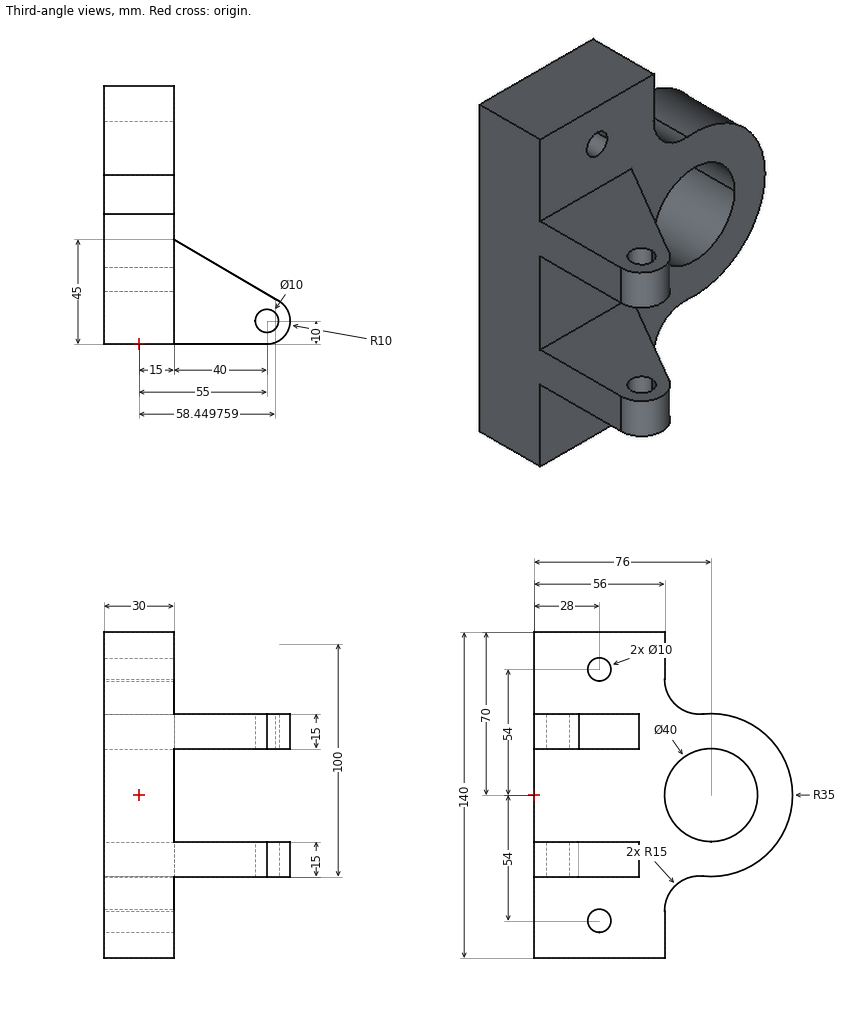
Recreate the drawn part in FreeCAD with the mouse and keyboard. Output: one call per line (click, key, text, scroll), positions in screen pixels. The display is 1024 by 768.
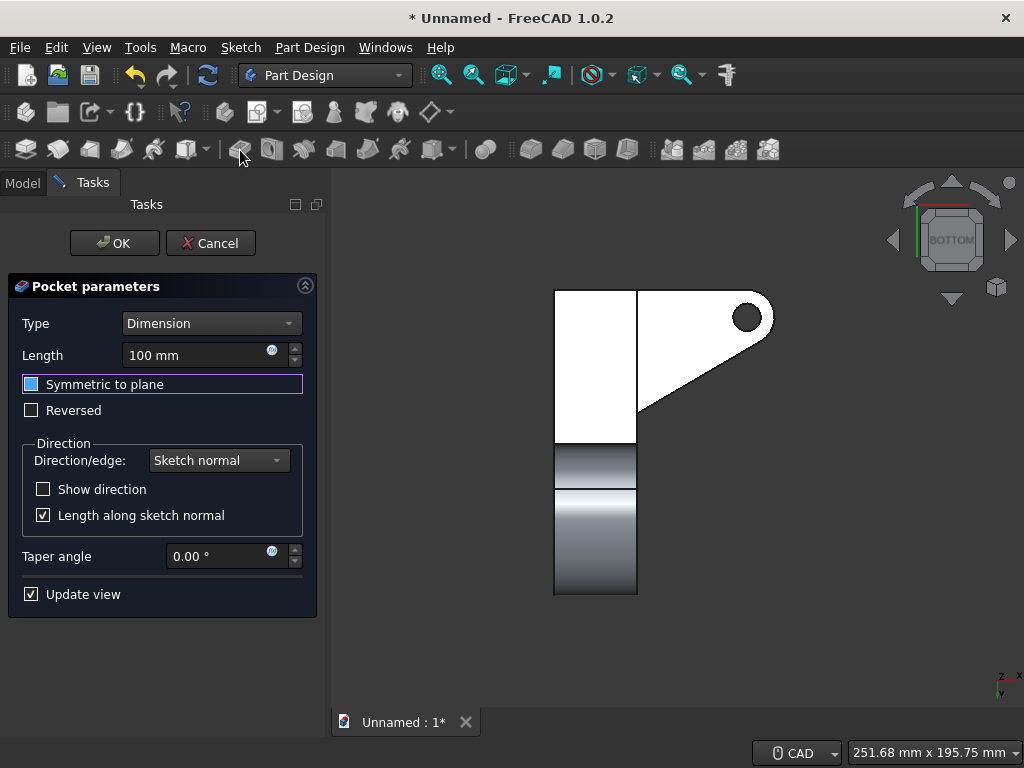
click(115, 243)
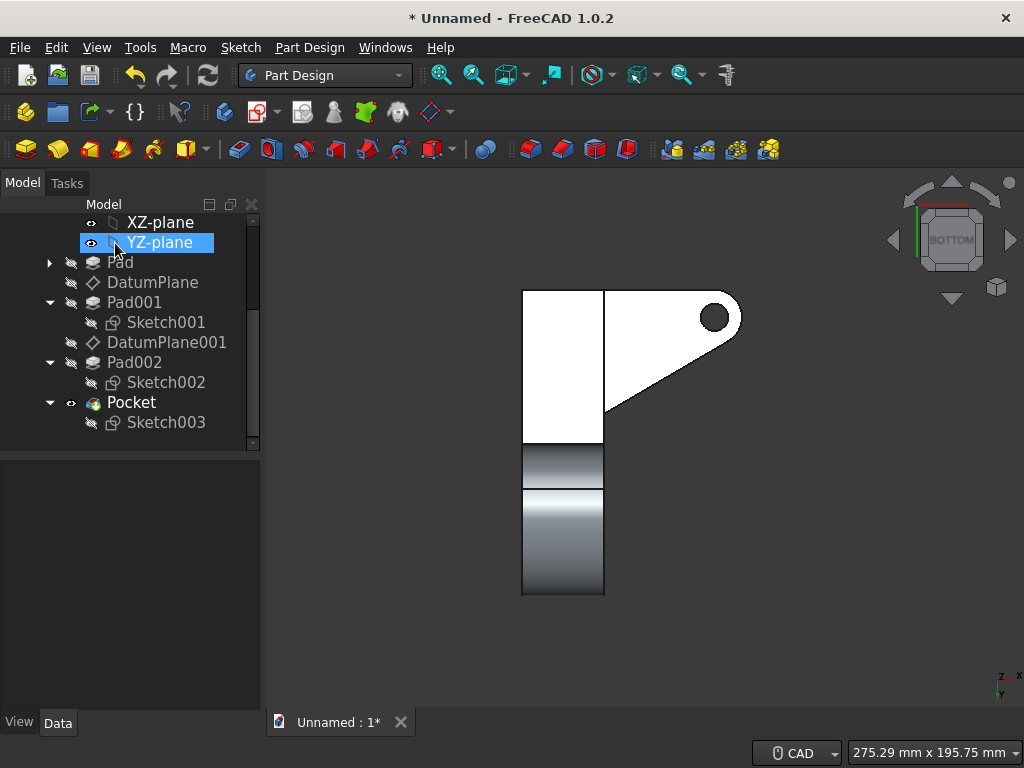
key(0)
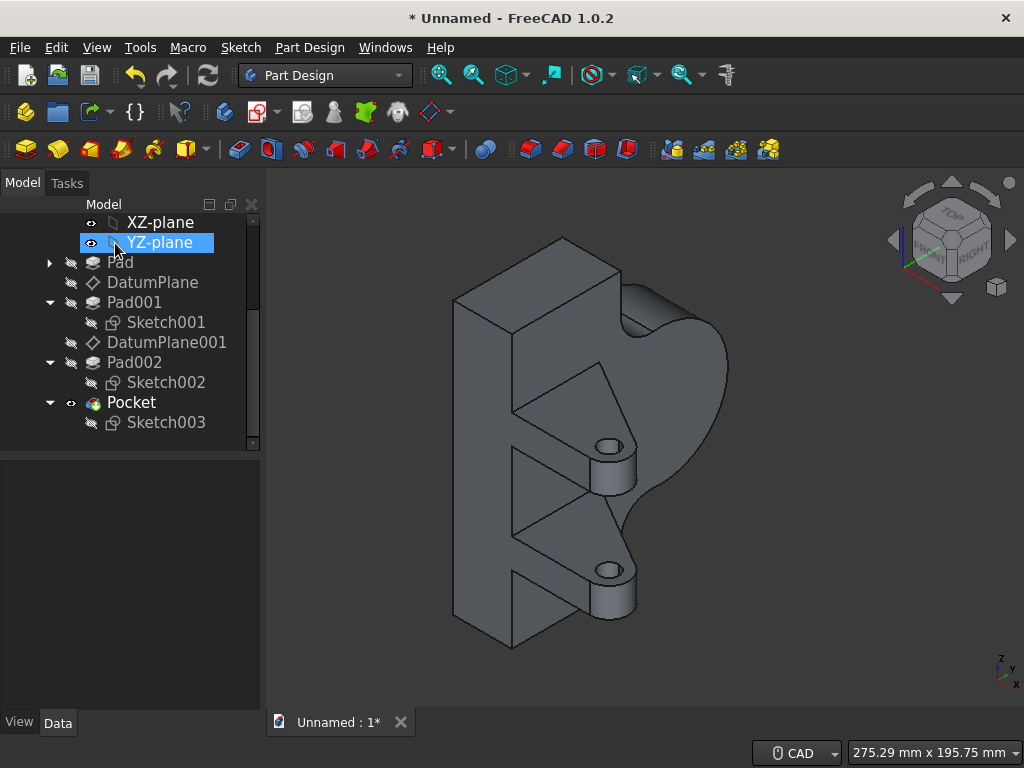
click(651, 410)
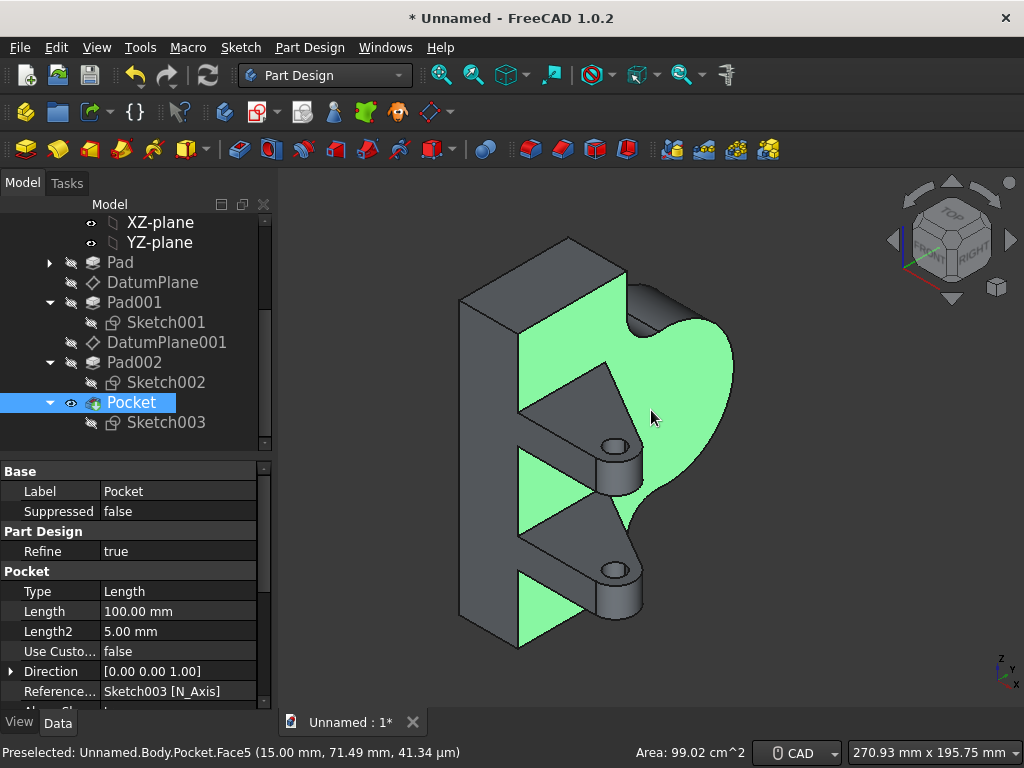
click(258, 112)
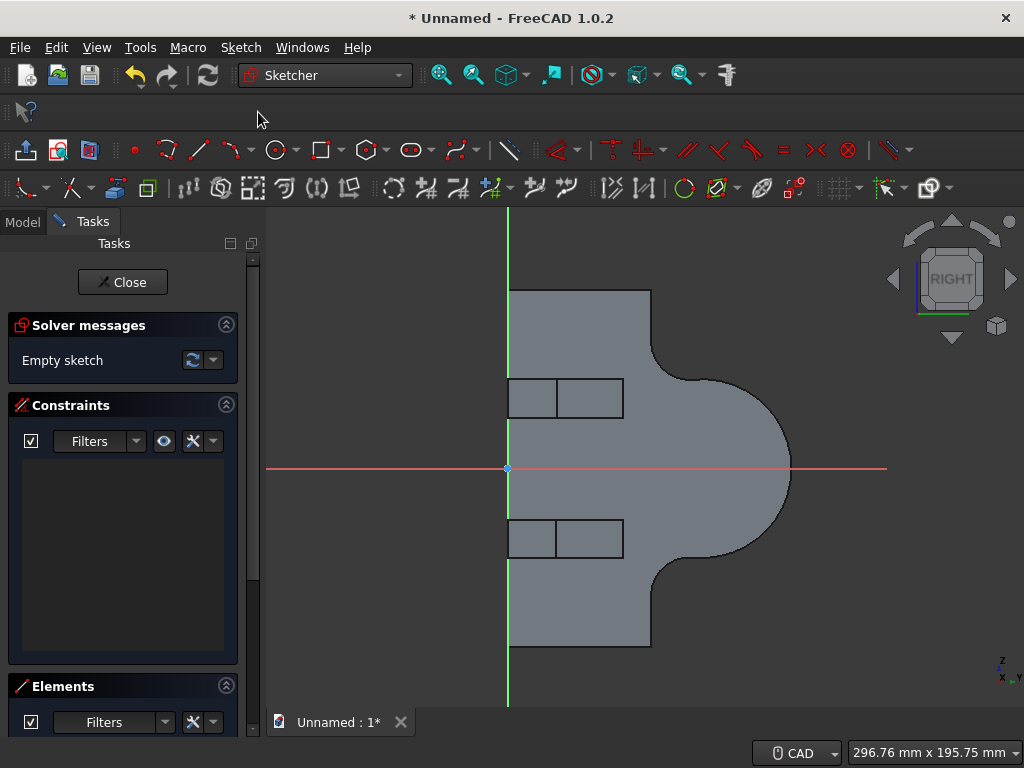
key(g)
key(c)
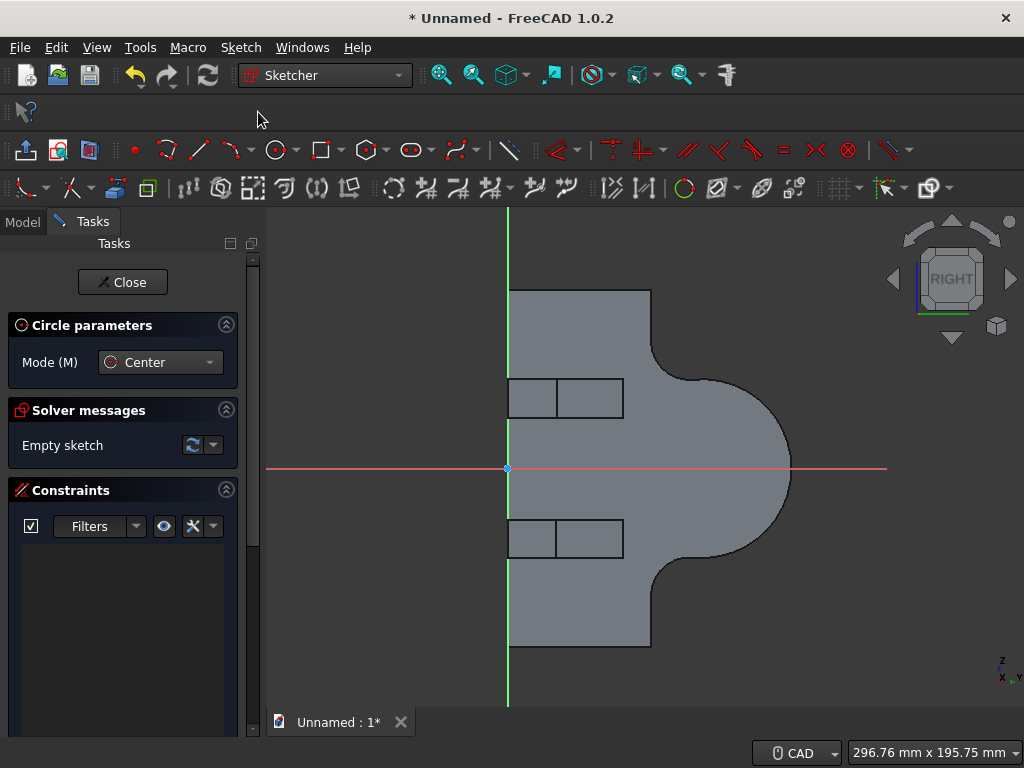
scroll(579, 331, up, 3)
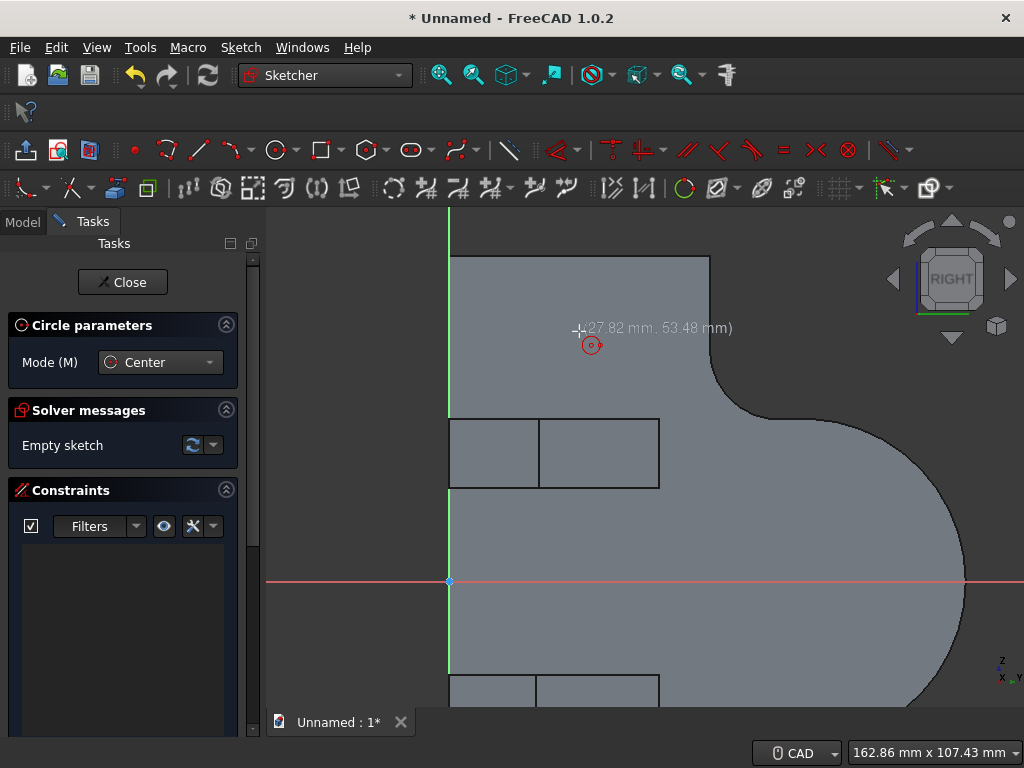
click(579, 330)
click(596, 314)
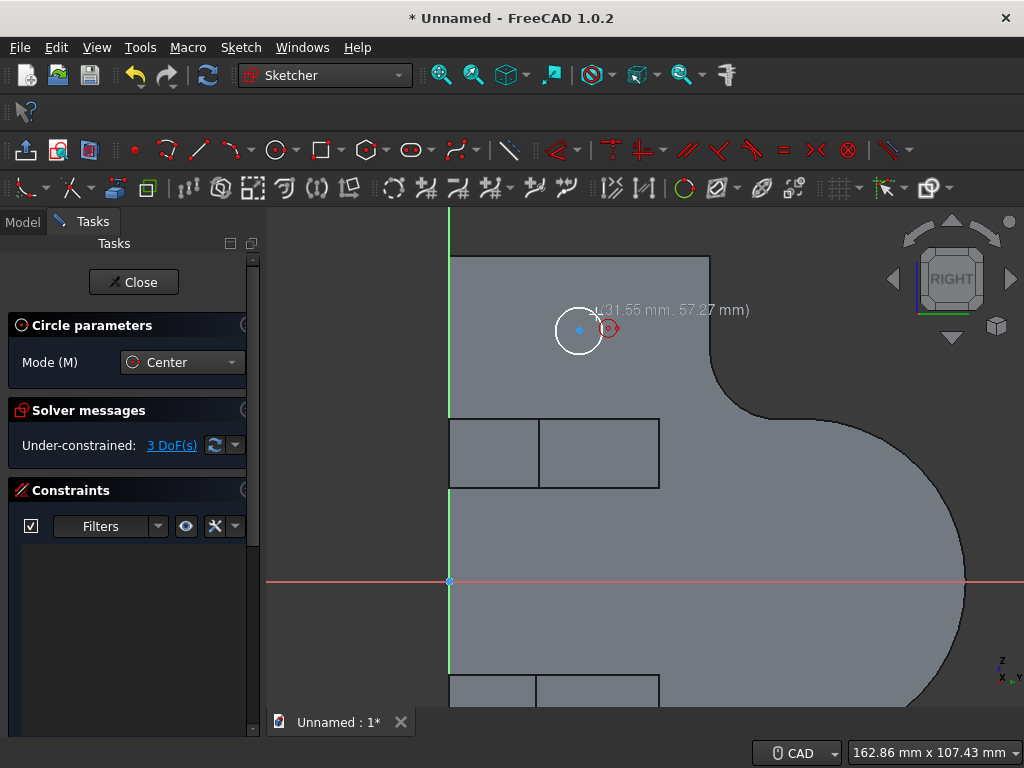
scroll(638, 306, down, 3)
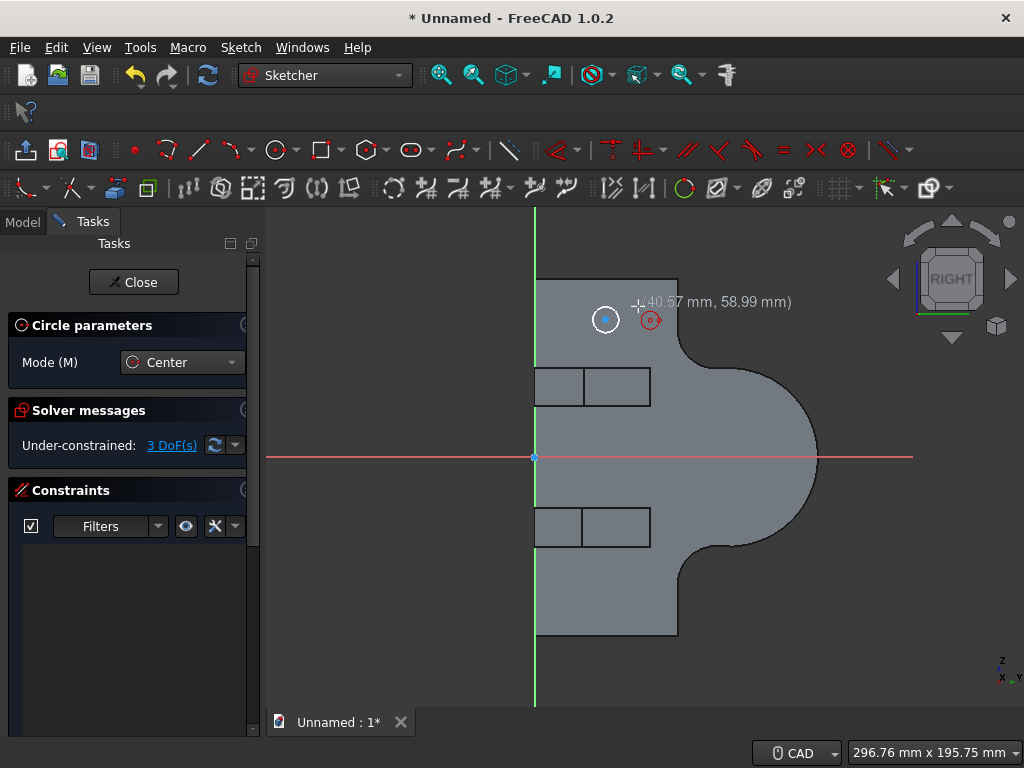
scroll(606, 595, up, 3)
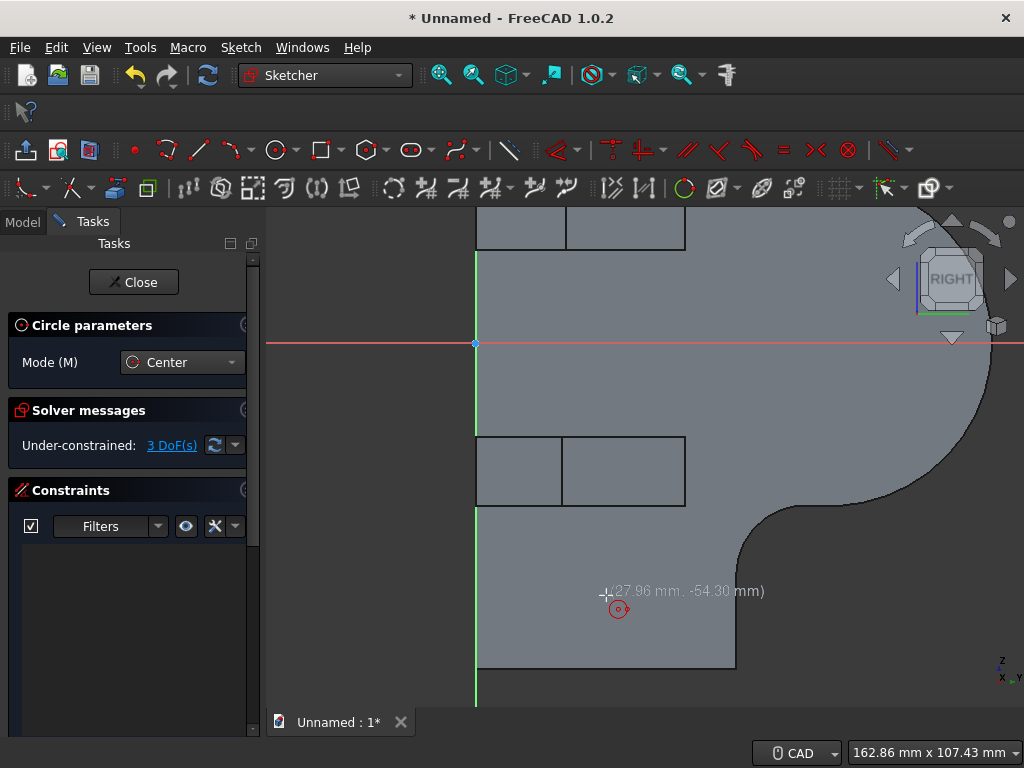
click(606, 595)
click(622, 578)
key(Escape)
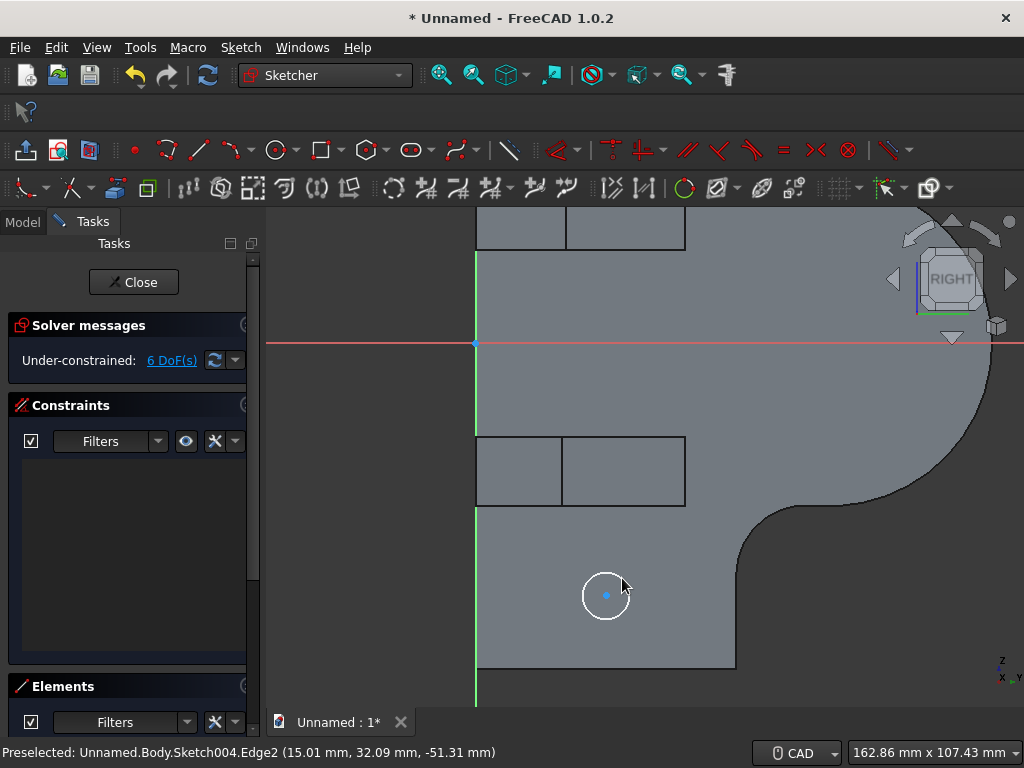
scroll(606, 595, down, 3)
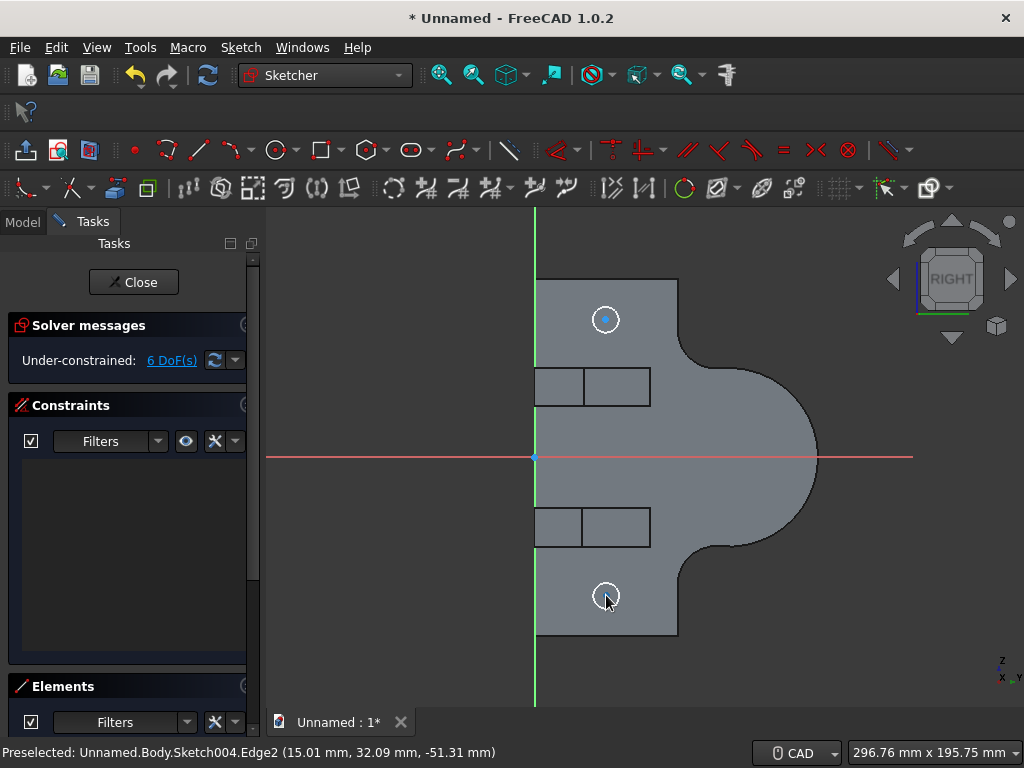
click(615, 311)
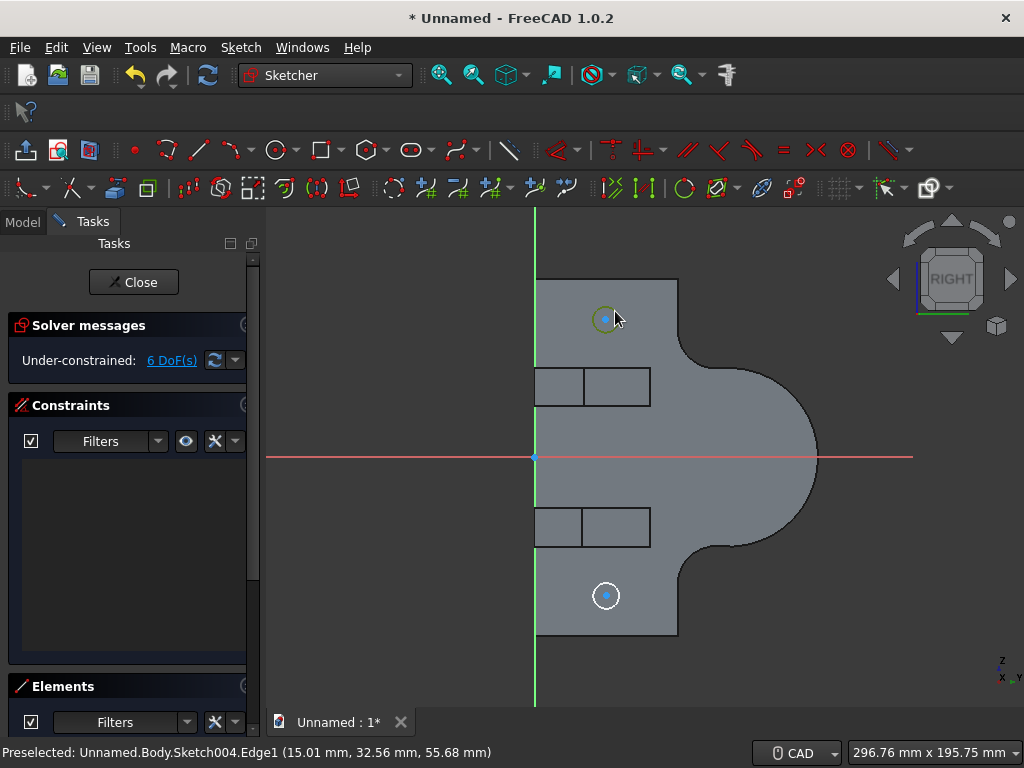
click(615, 587)